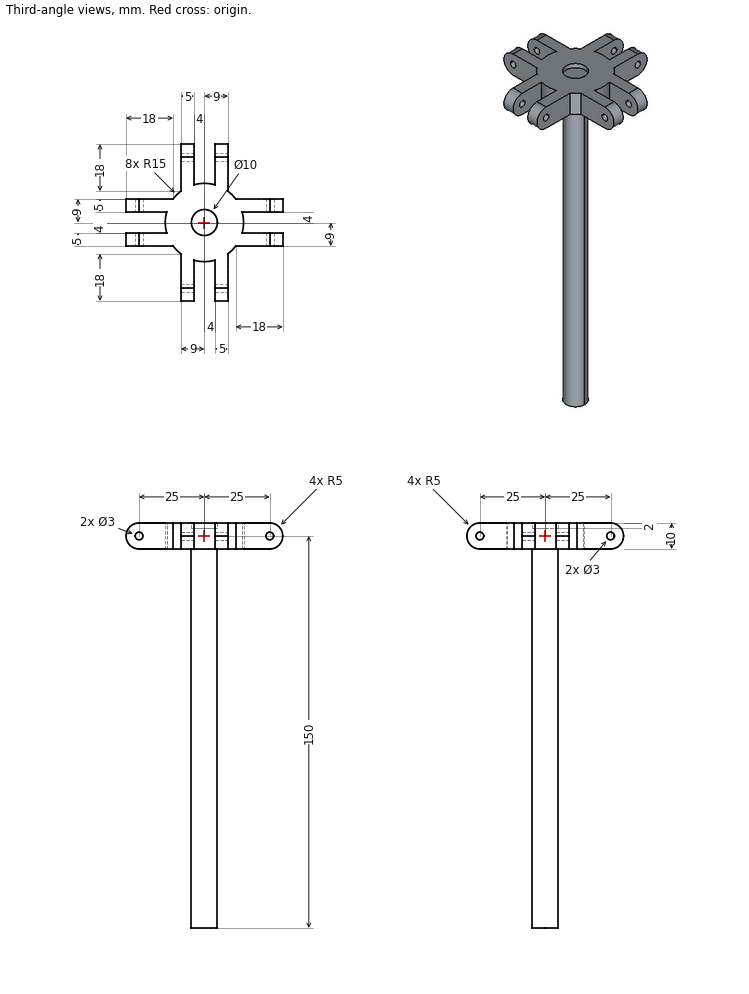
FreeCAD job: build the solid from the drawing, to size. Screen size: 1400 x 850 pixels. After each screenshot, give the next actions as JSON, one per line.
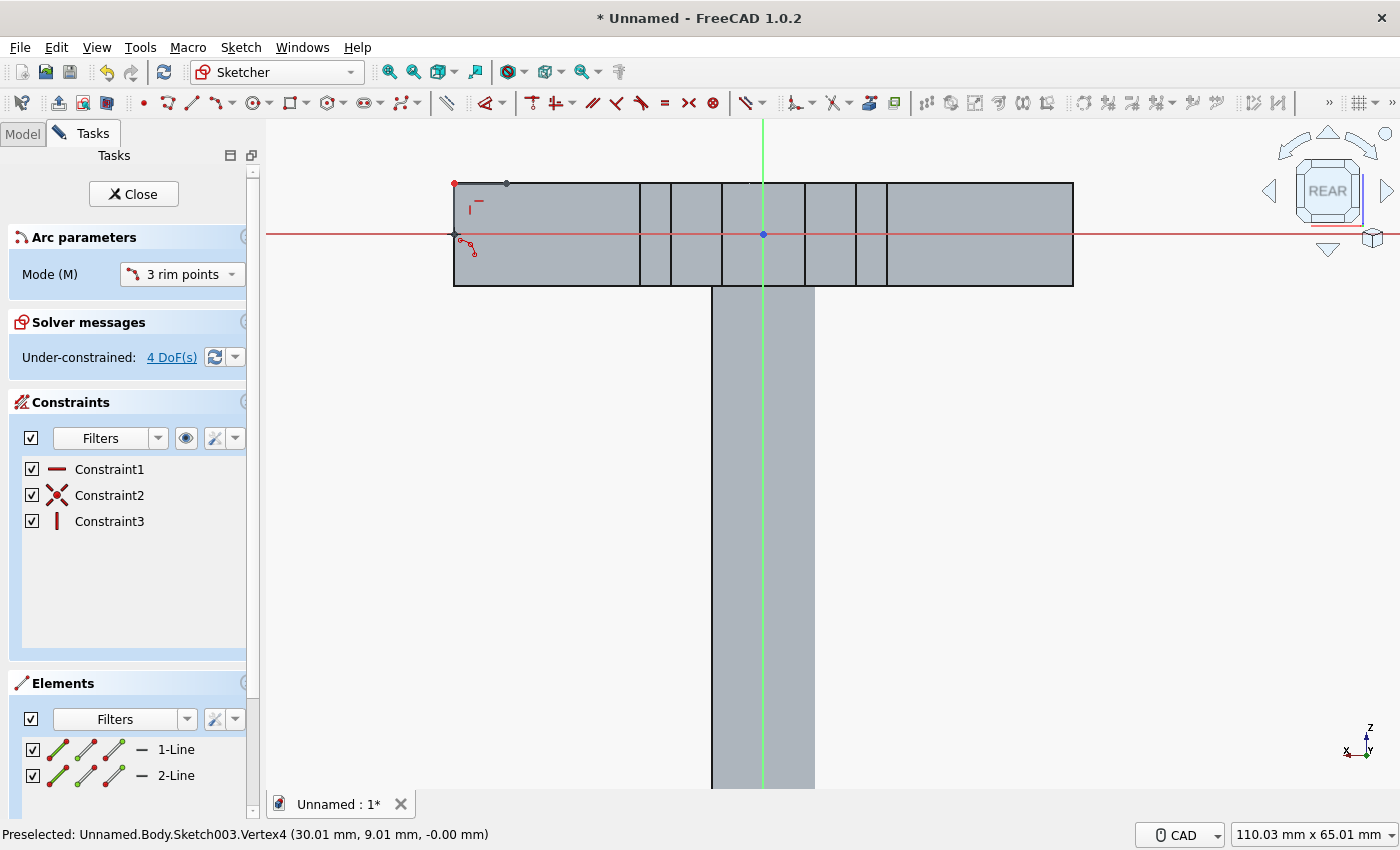
{"action": "left_click", "coordinate": [454, 234]}
{"action": "left_click", "coordinate": [506, 184]}
{"action": "left_click", "coordinate": [469, 198]}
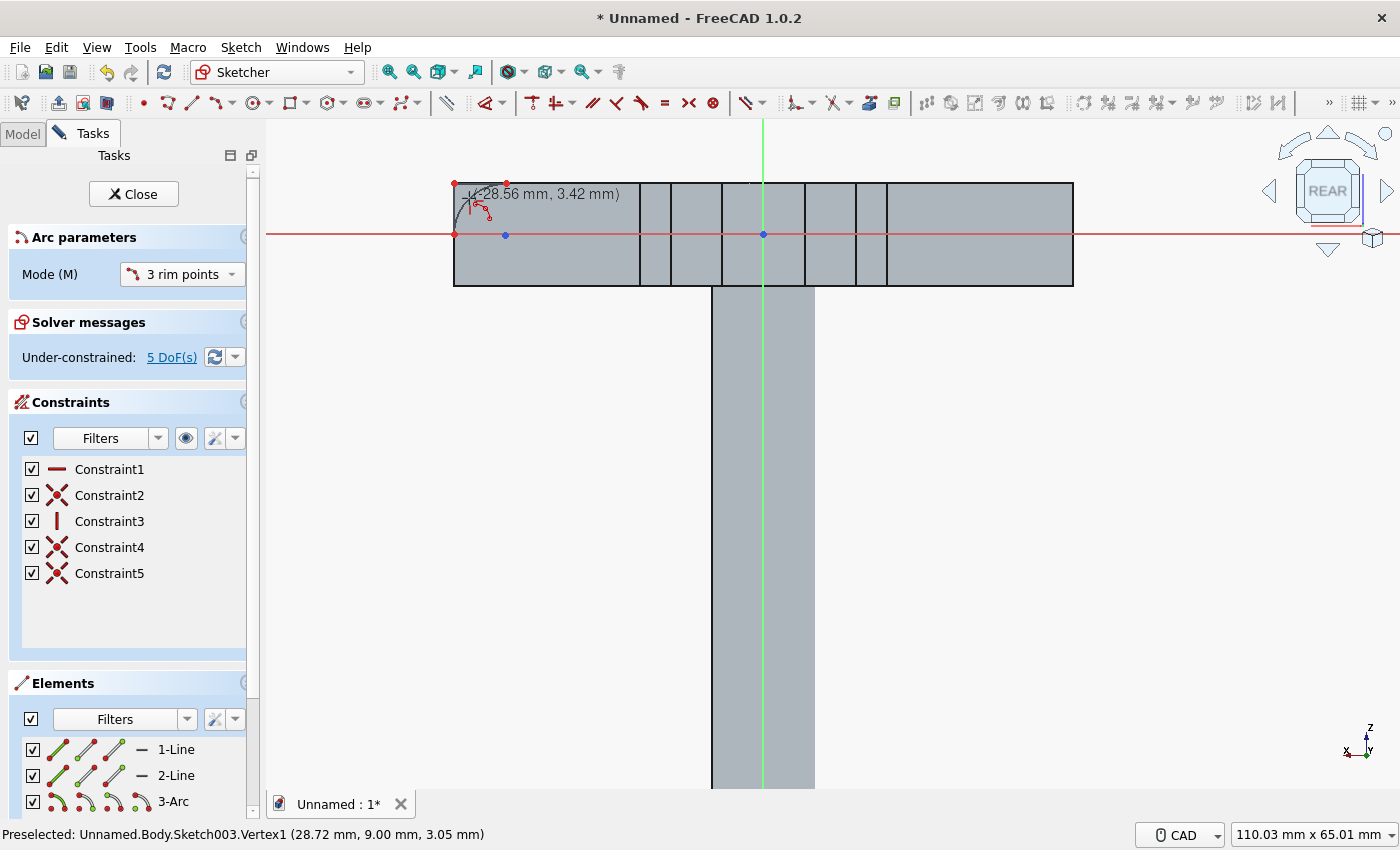
{"action": "key", "text": "g m"}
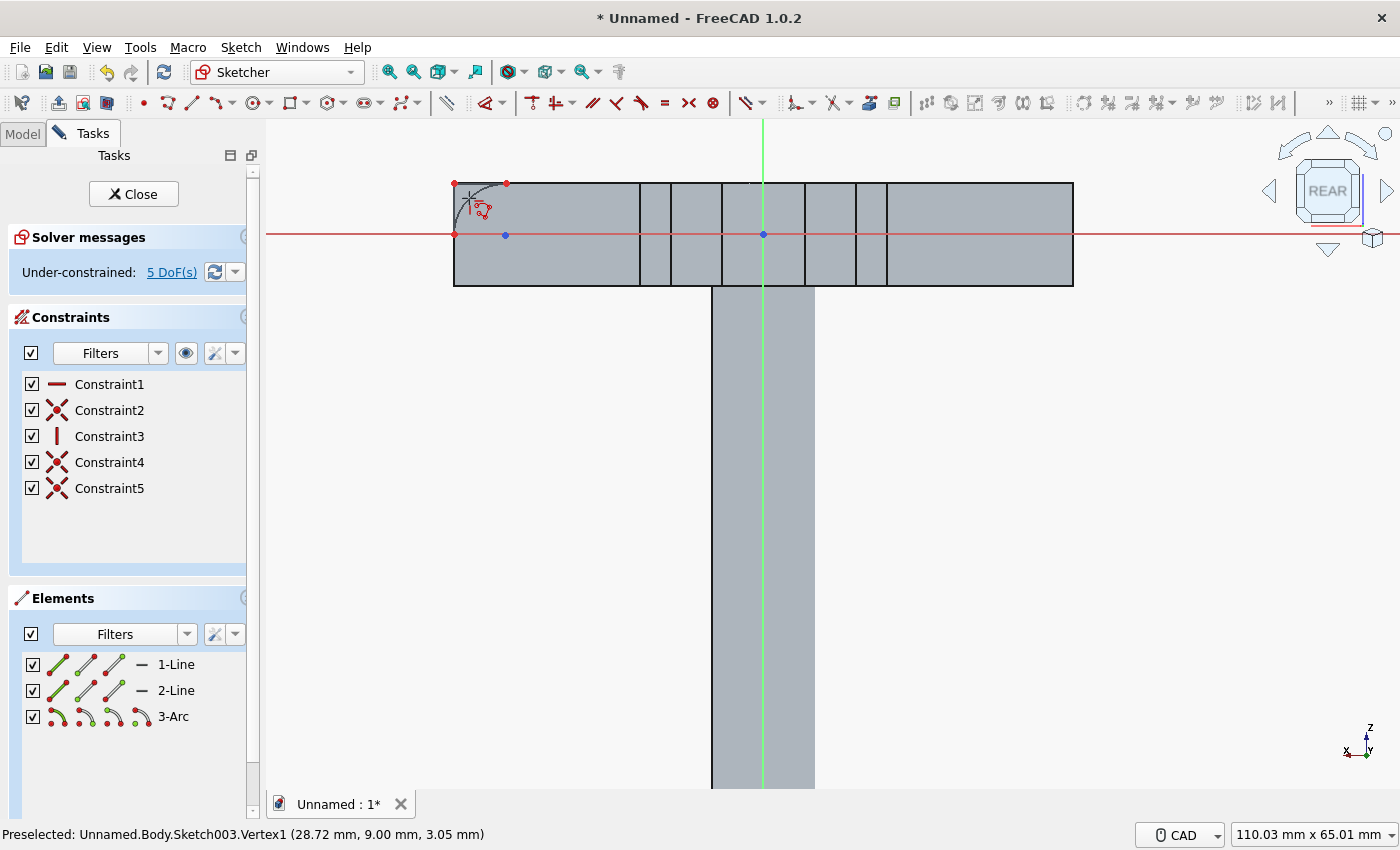
{"action": "left_click", "coordinate": [454, 234]}
{"action": "left_click", "coordinate": [454, 286]}
{"action": "left_click", "coordinate": [506, 286]}
{"action": "right_click", "coordinate": [506, 286]}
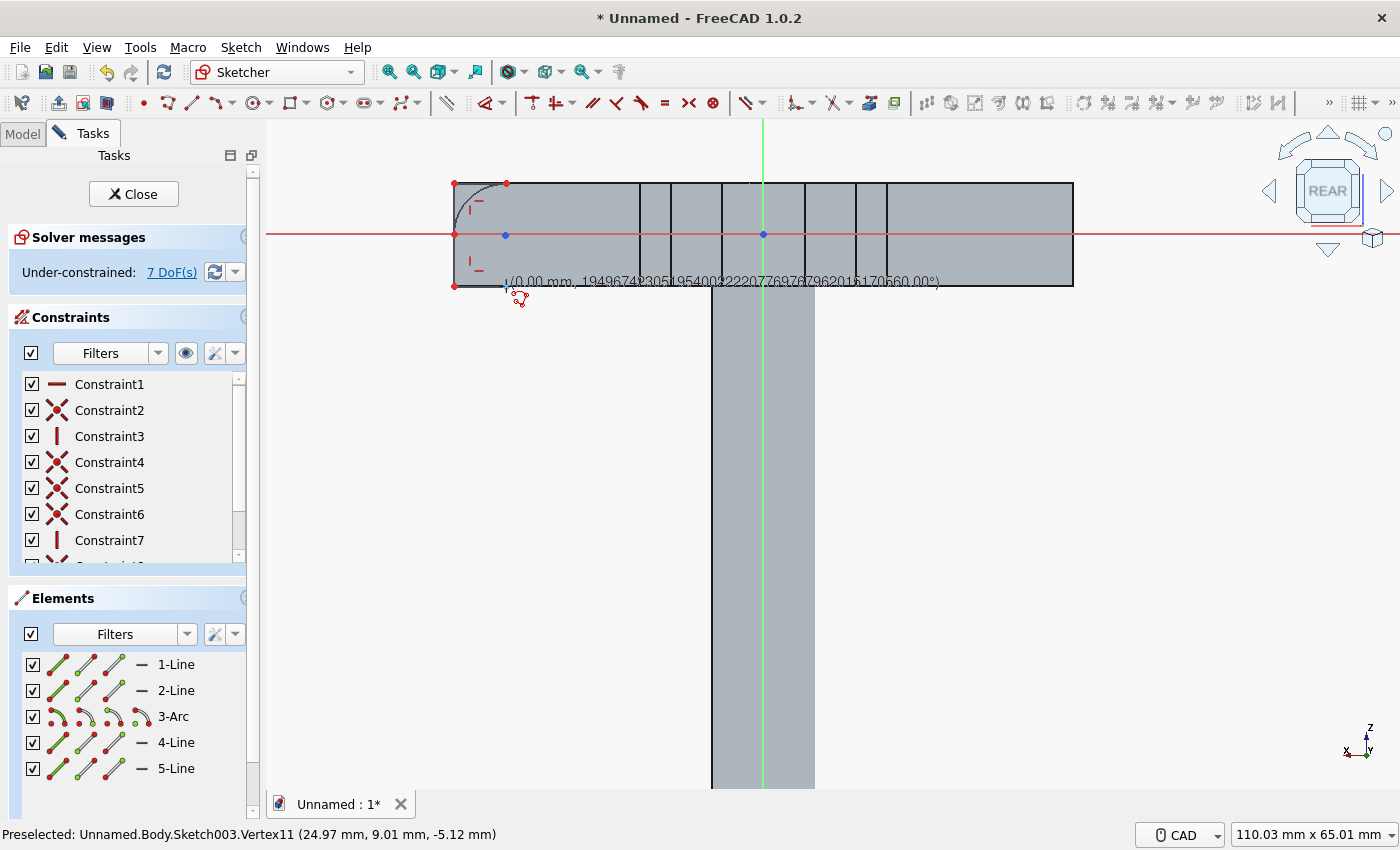
{"action": "key", "text": "g 3 a"}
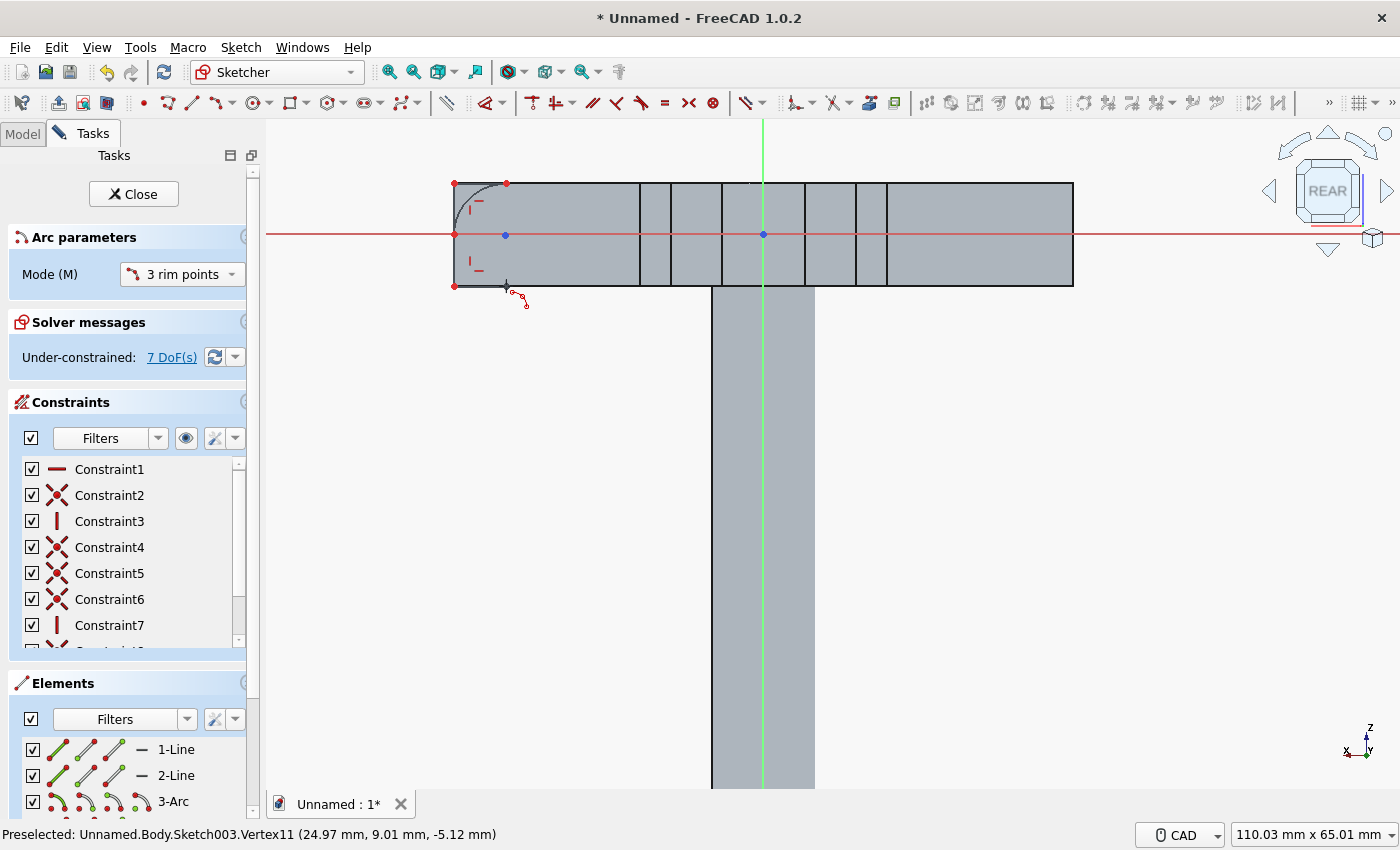
{"action": "left_click", "coordinate": [506, 287]}
{"action": "left_click", "coordinate": [454, 234]}
{"action": "left_click", "coordinate": [469, 271]}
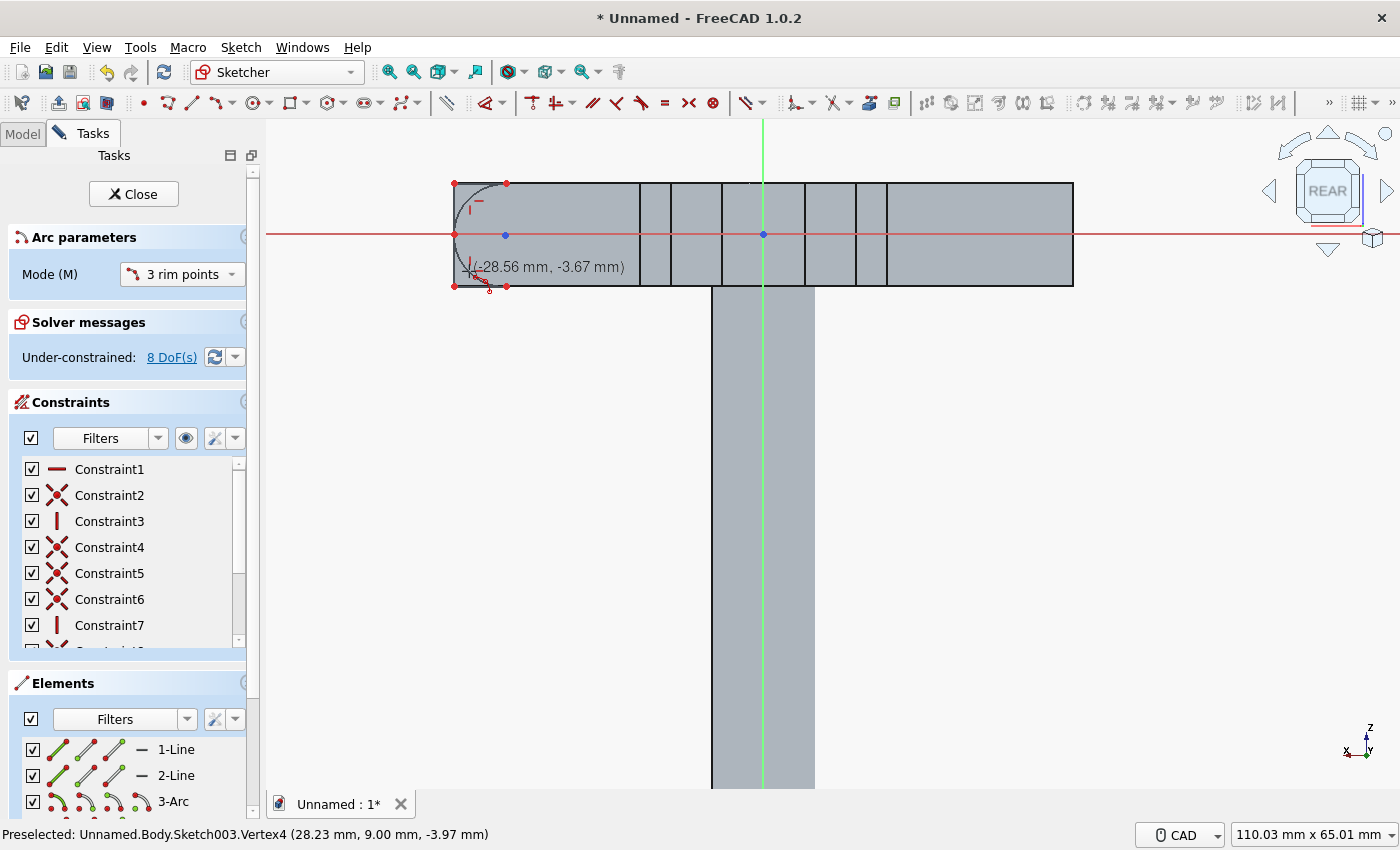
{"action": "key", "text": "g m"}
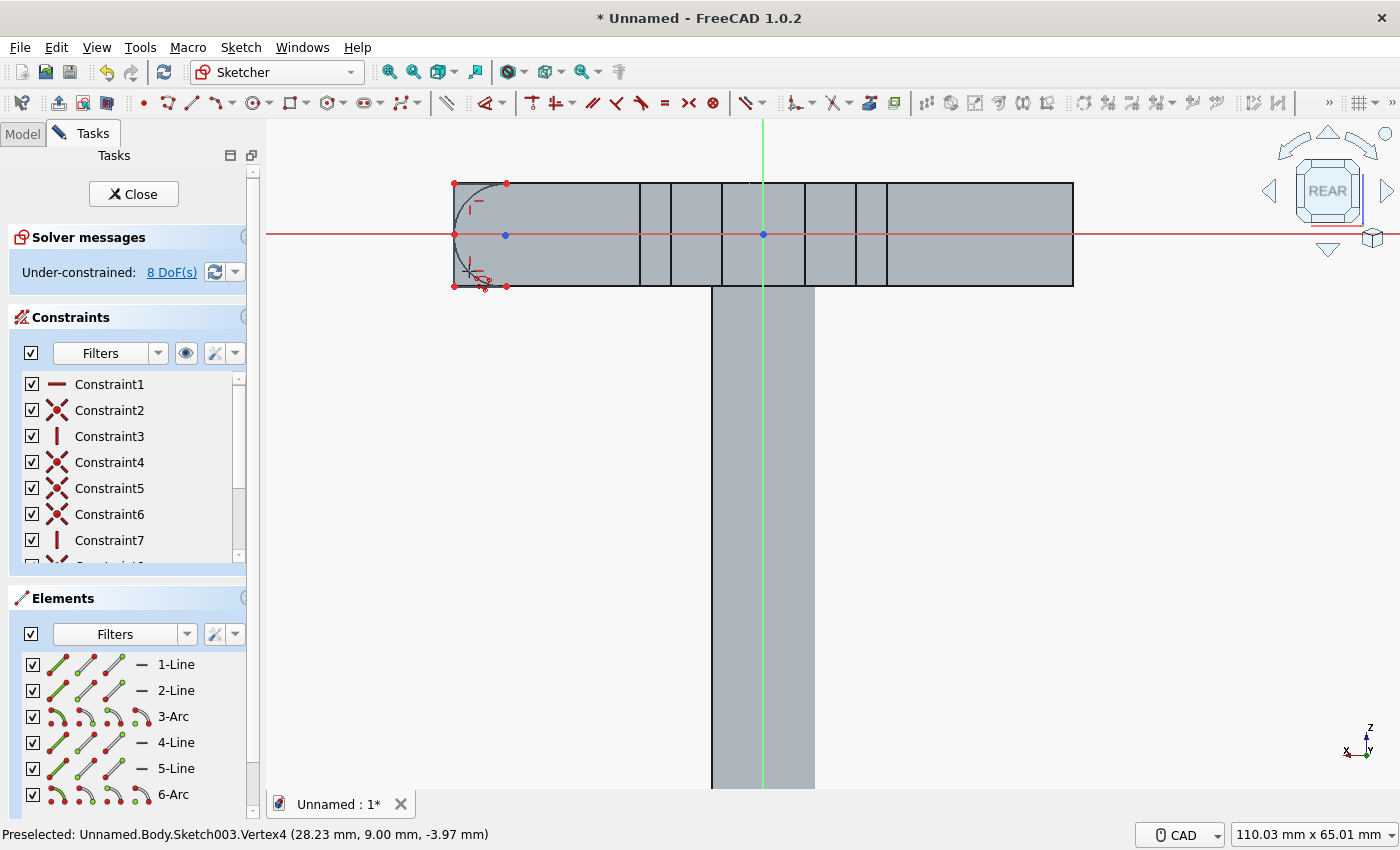
{"action": "left_click", "coordinate": [1073, 234]}
{"action": "left_click", "coordinate": [1073, 183]}
{"action": "left_click", "coordinate": [1021, 183]}
{"action": "right_click", "coordinate": [1021, 183]}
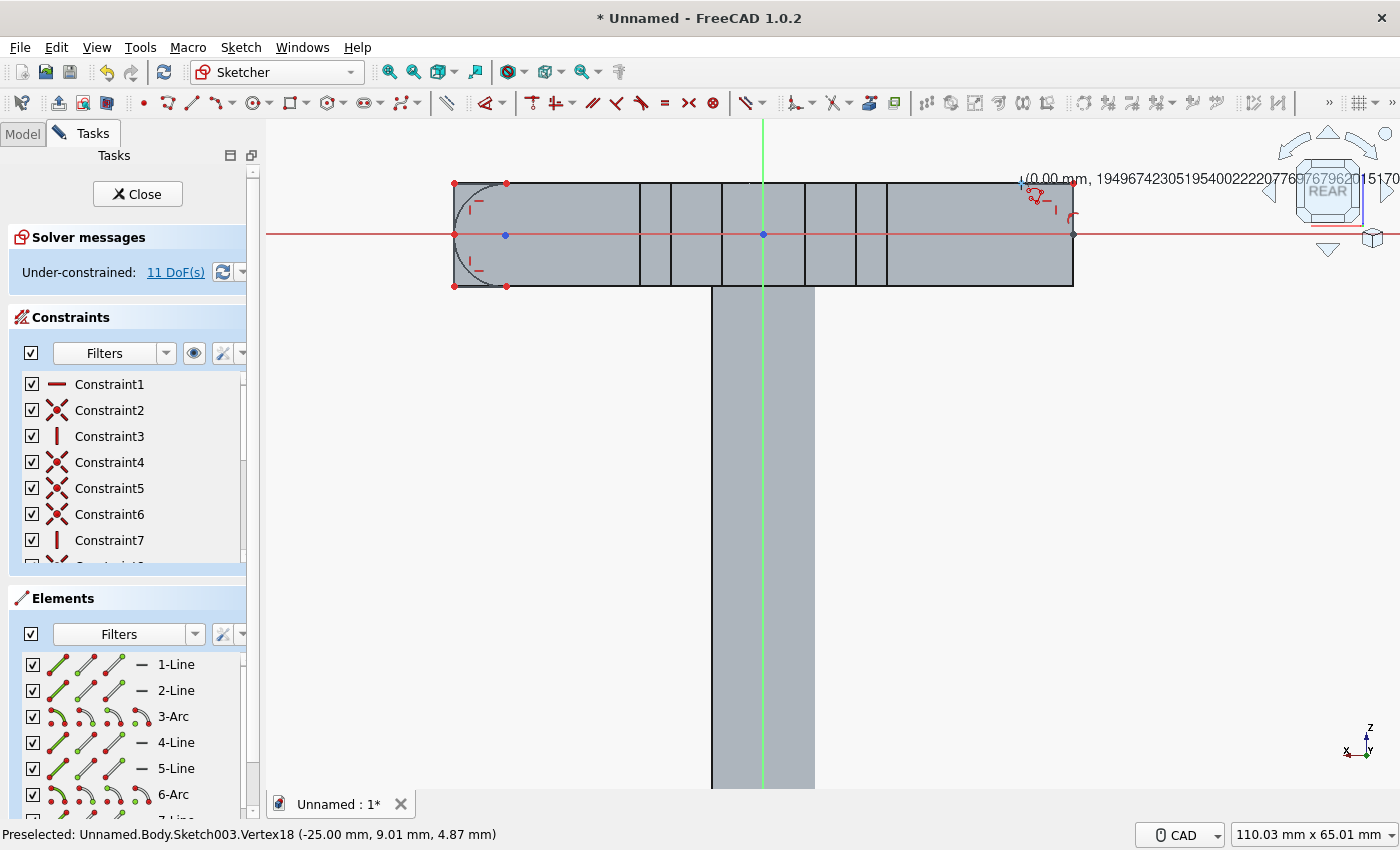
{"action": "key", "text": "g 3 a"}